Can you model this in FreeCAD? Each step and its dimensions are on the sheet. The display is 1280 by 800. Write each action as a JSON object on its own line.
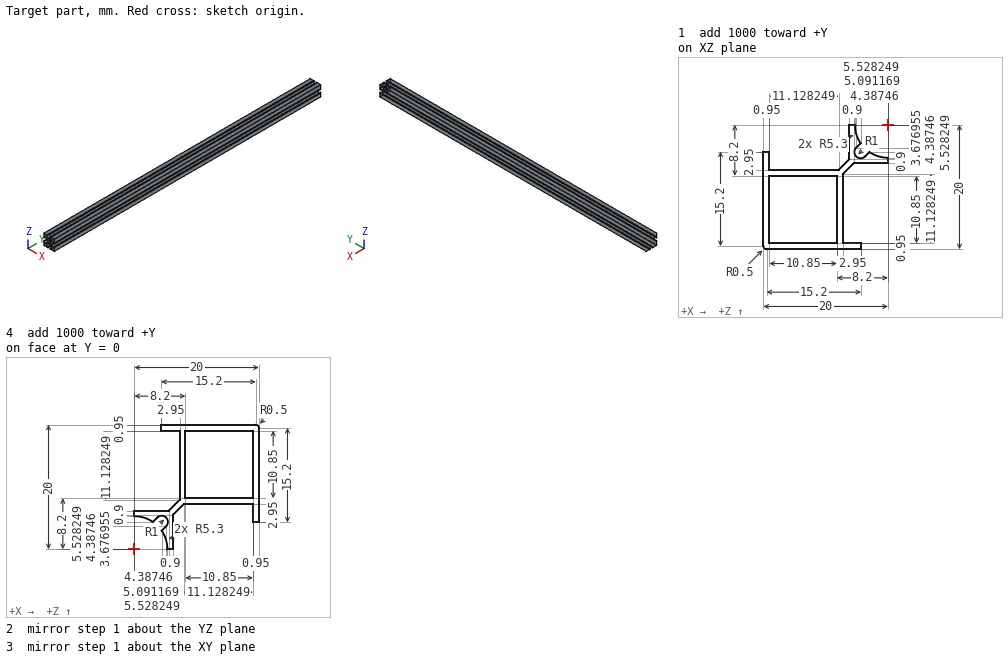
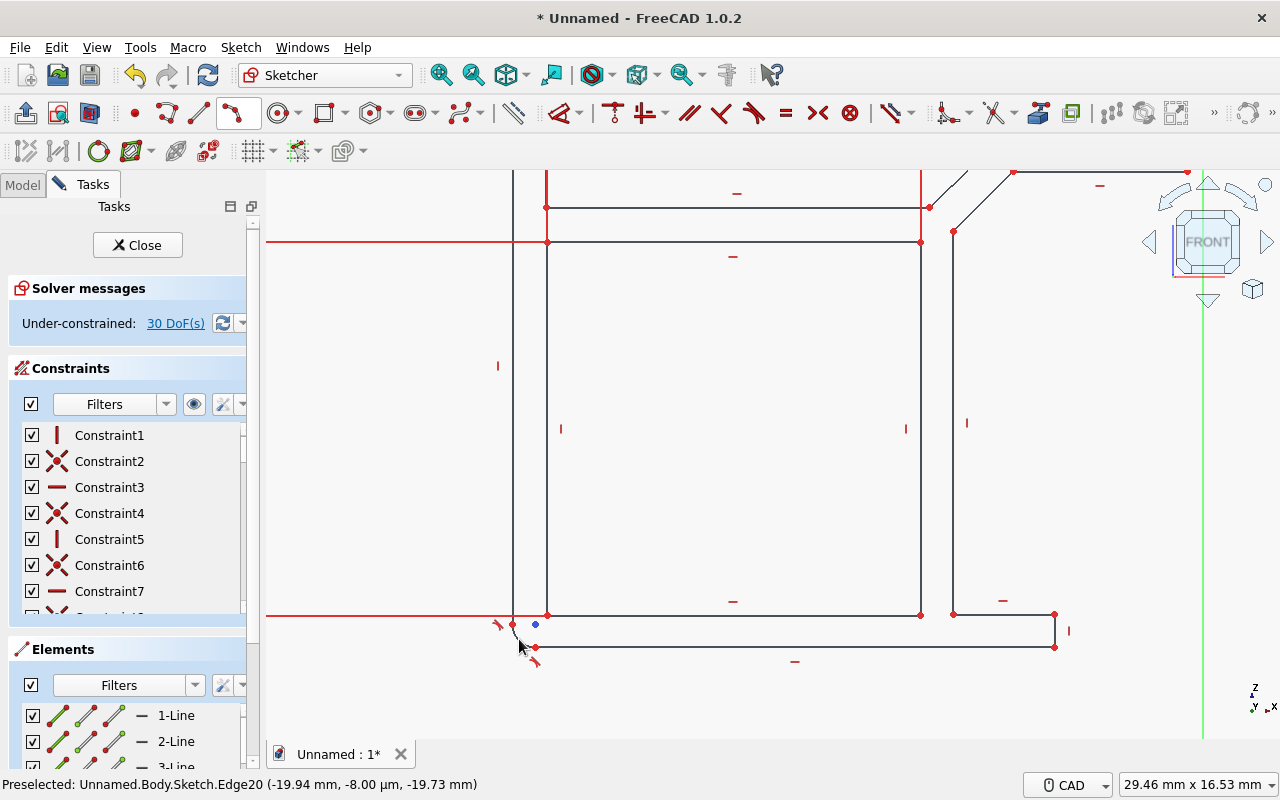
{"action": "scroll", "coordinate": [517, 641], "scroll_direction": "down", "scroll_amount": 3}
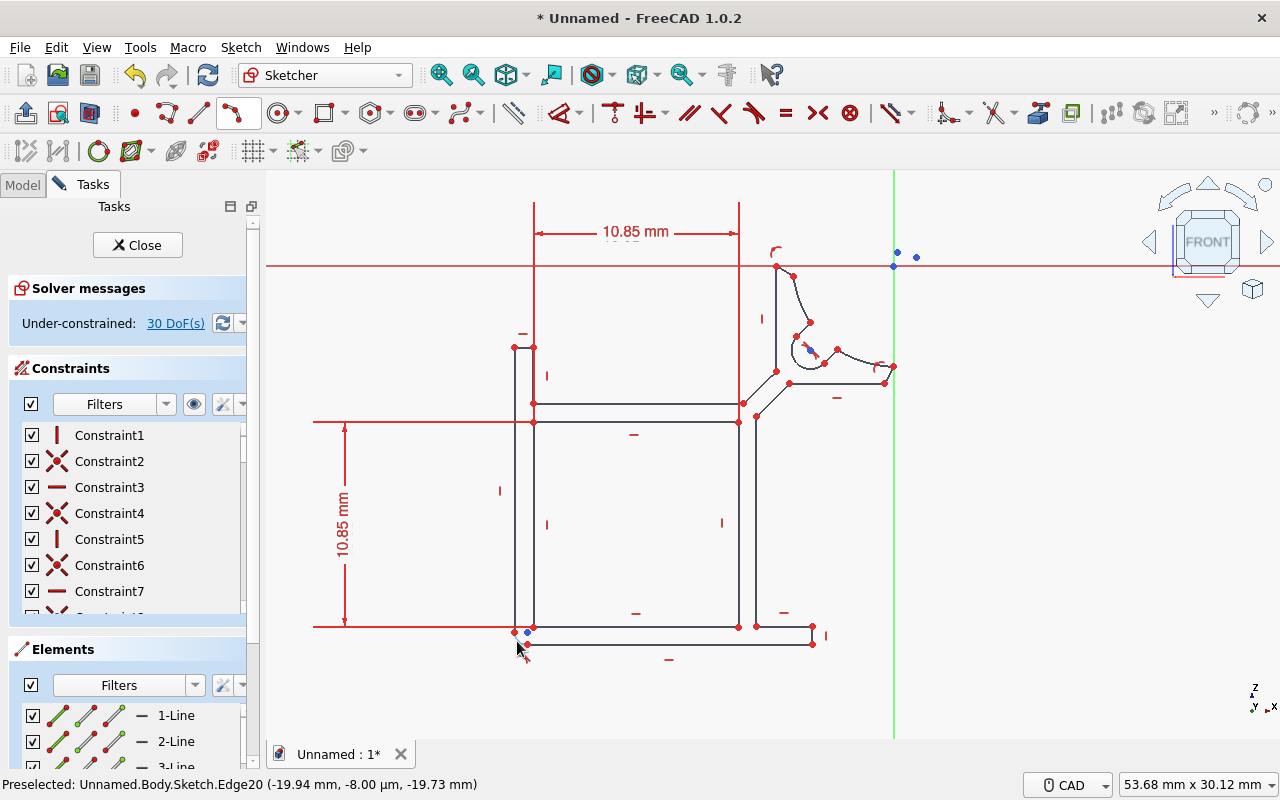
{"action": "scroll", "coordinate": [788, 273], "scroll_direction": "up", "scroll_amount": 5}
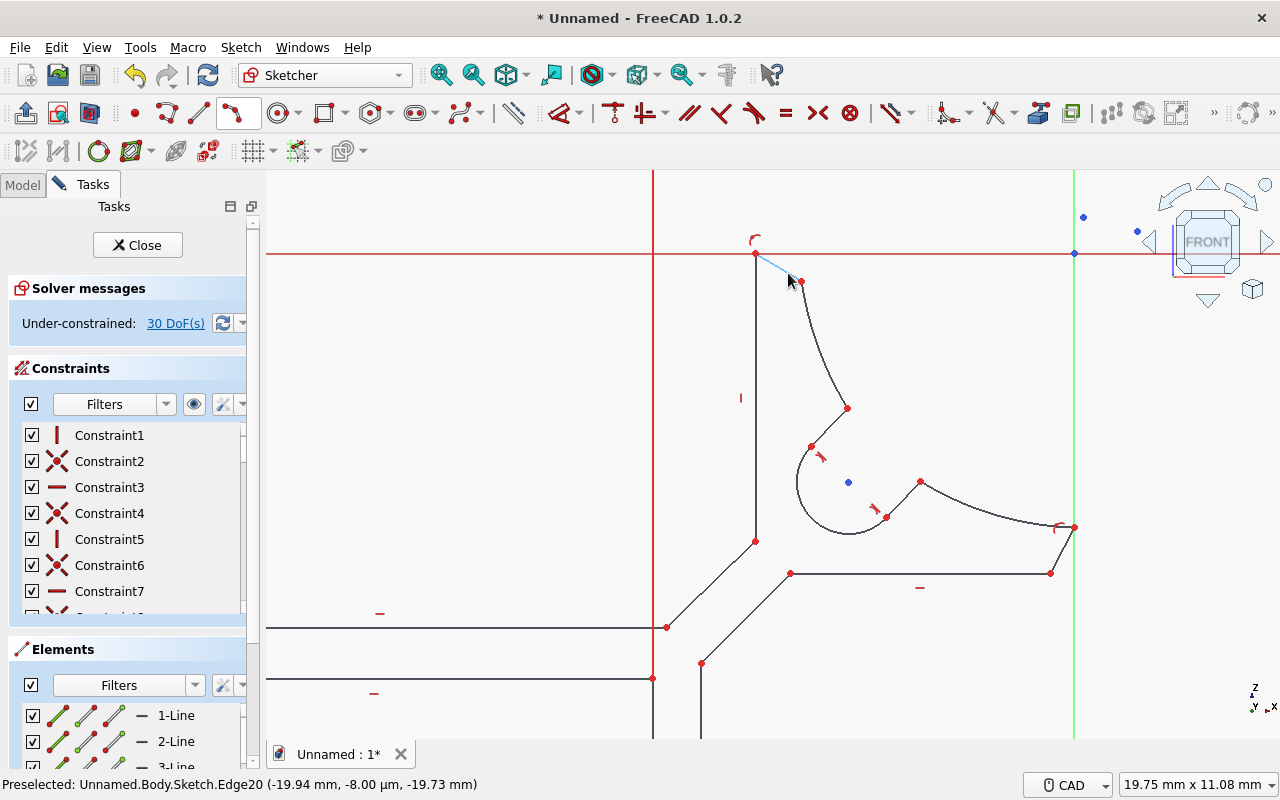
{"action": "left_click", "coordinate": [788, 273]}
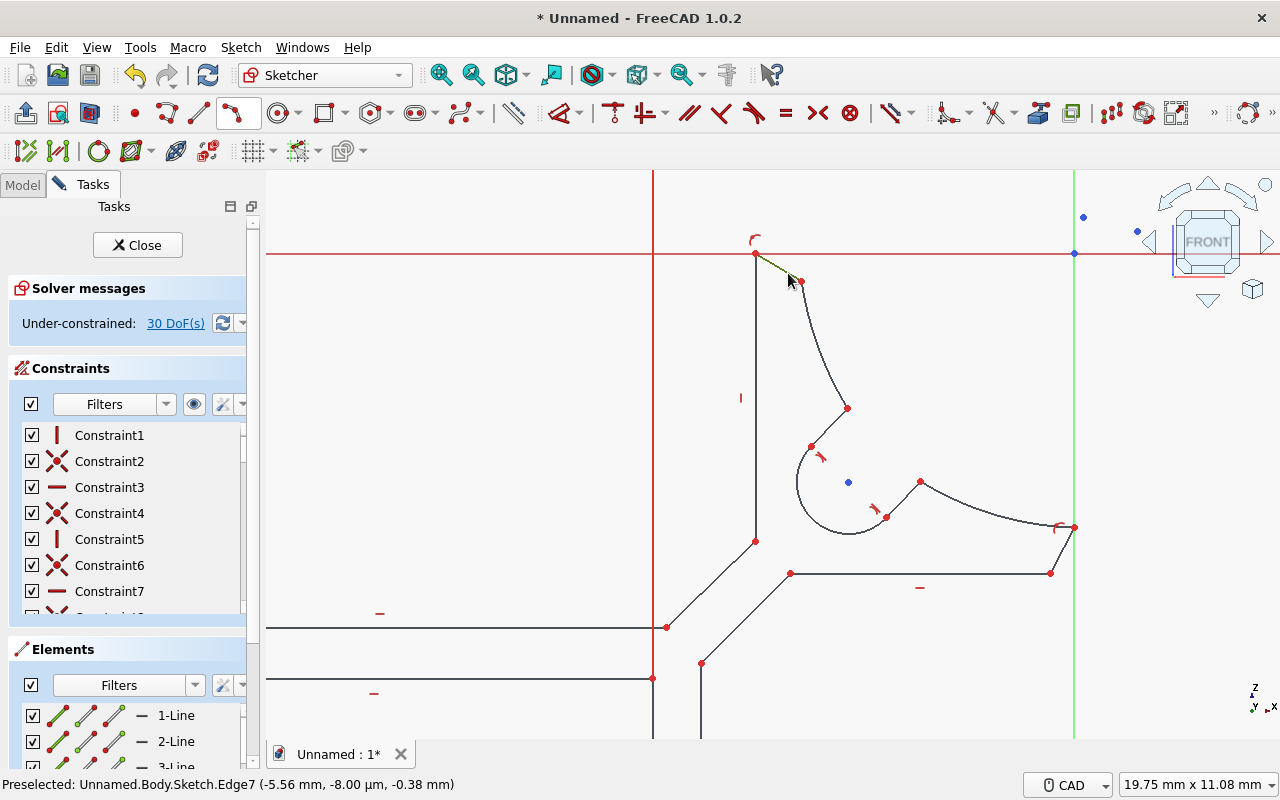
{"action": "left_click", "coordinate": [668, 114]}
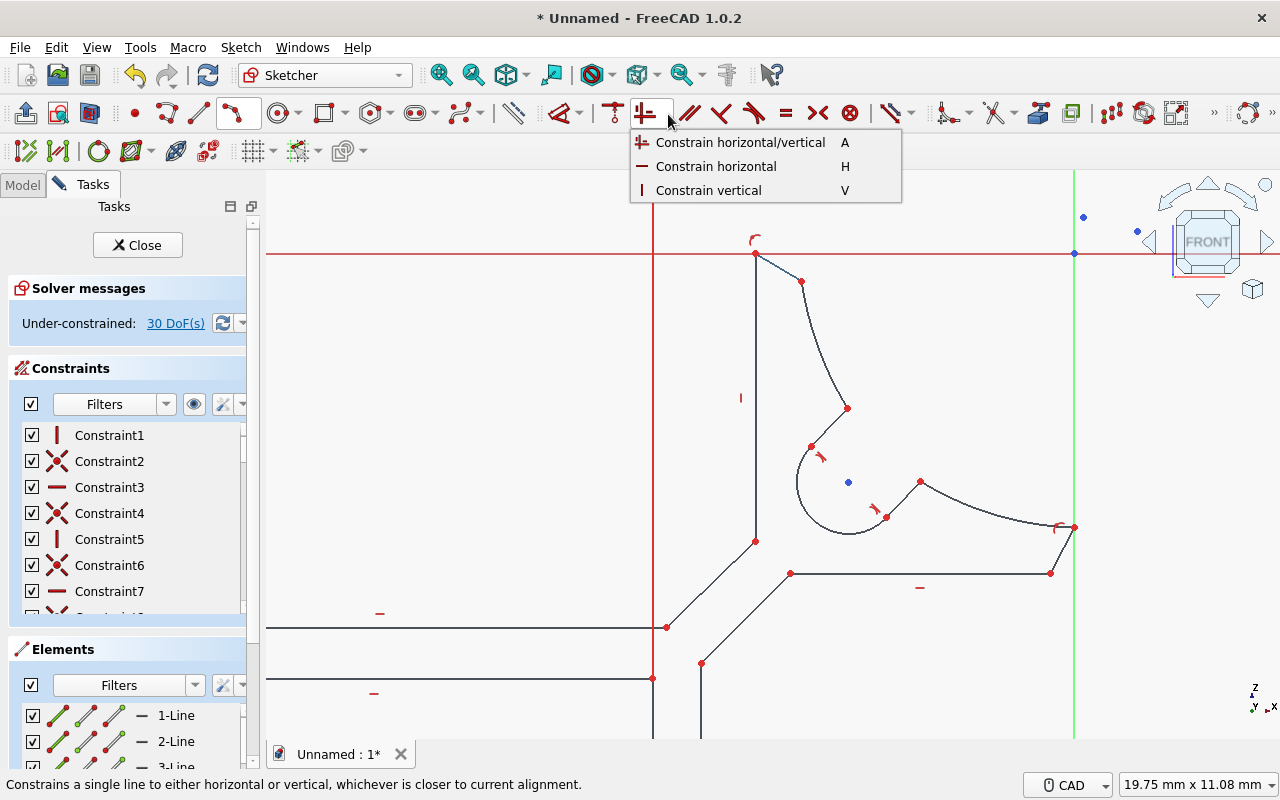
{"action": "left_click", "coordinate": [766, 166]}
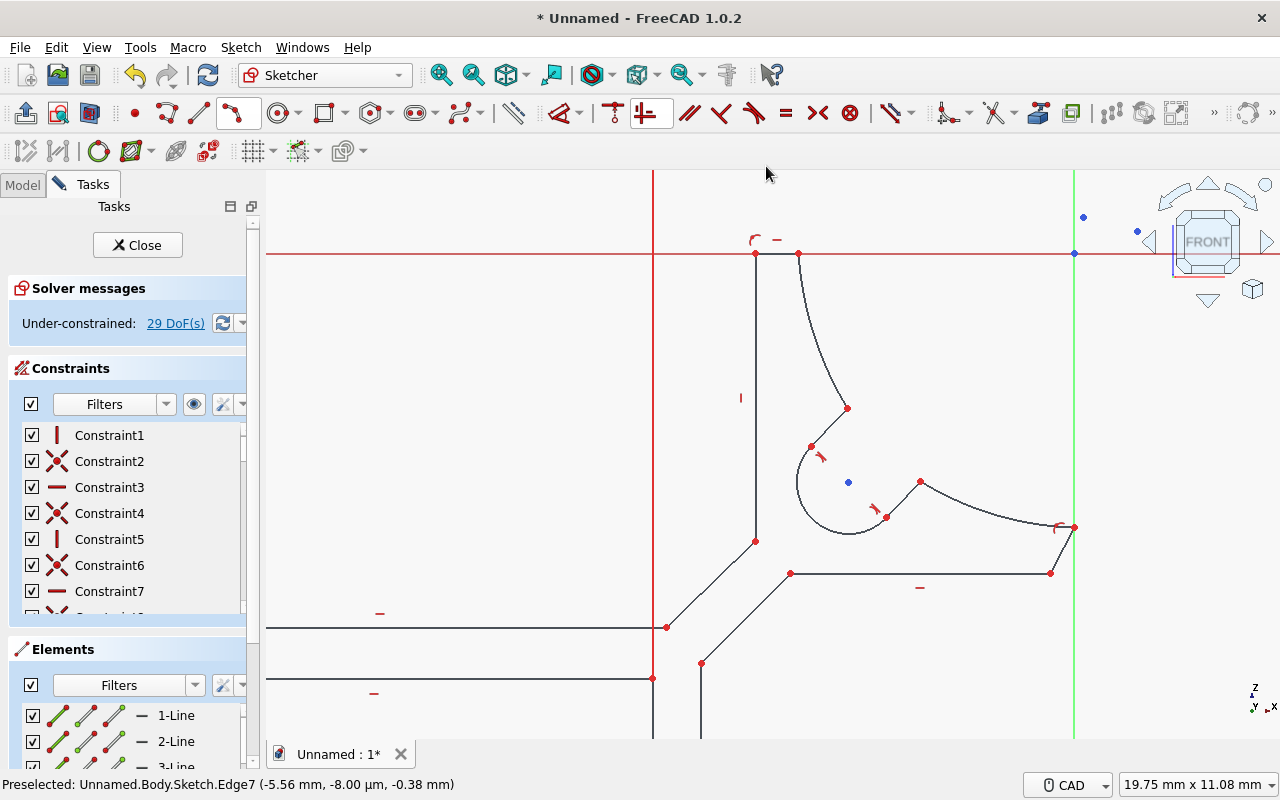
{"action": "left_click", "coordinate": [1058, 560]}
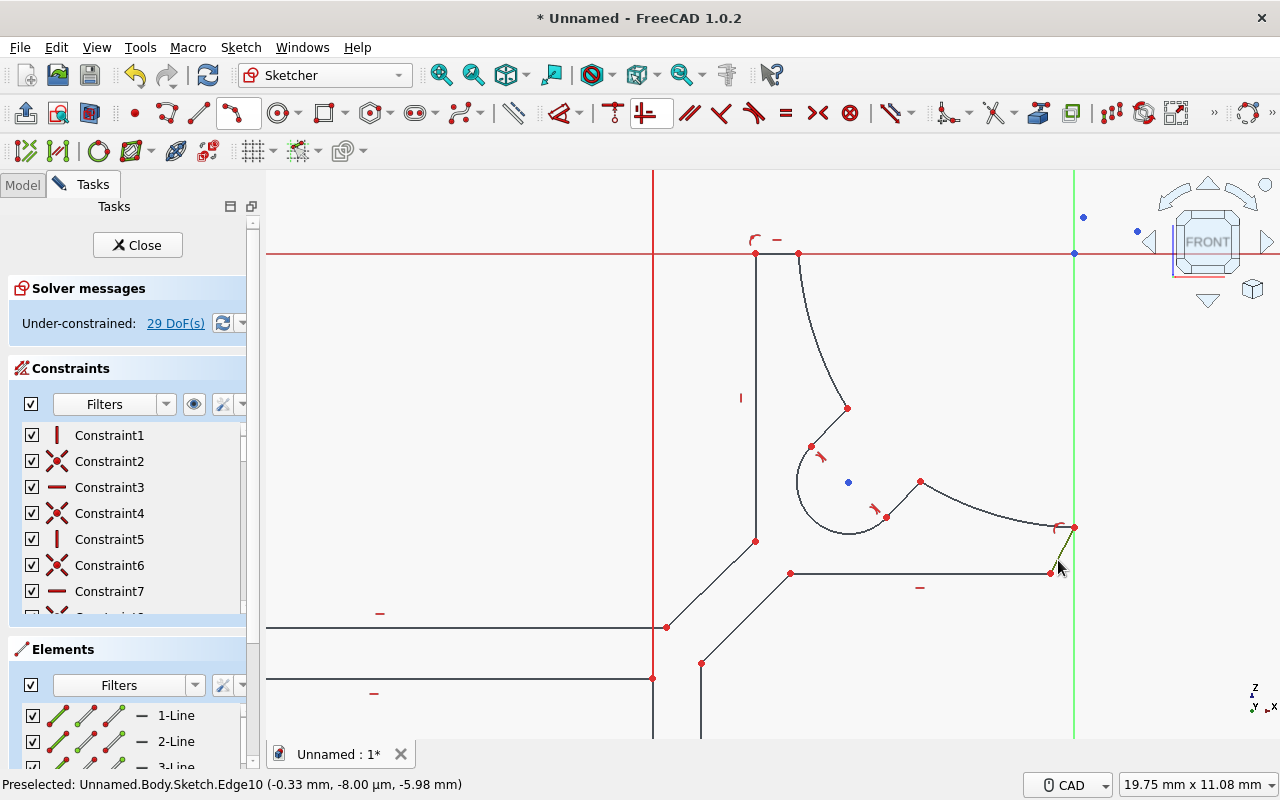
{"action": "key", "text": "v"}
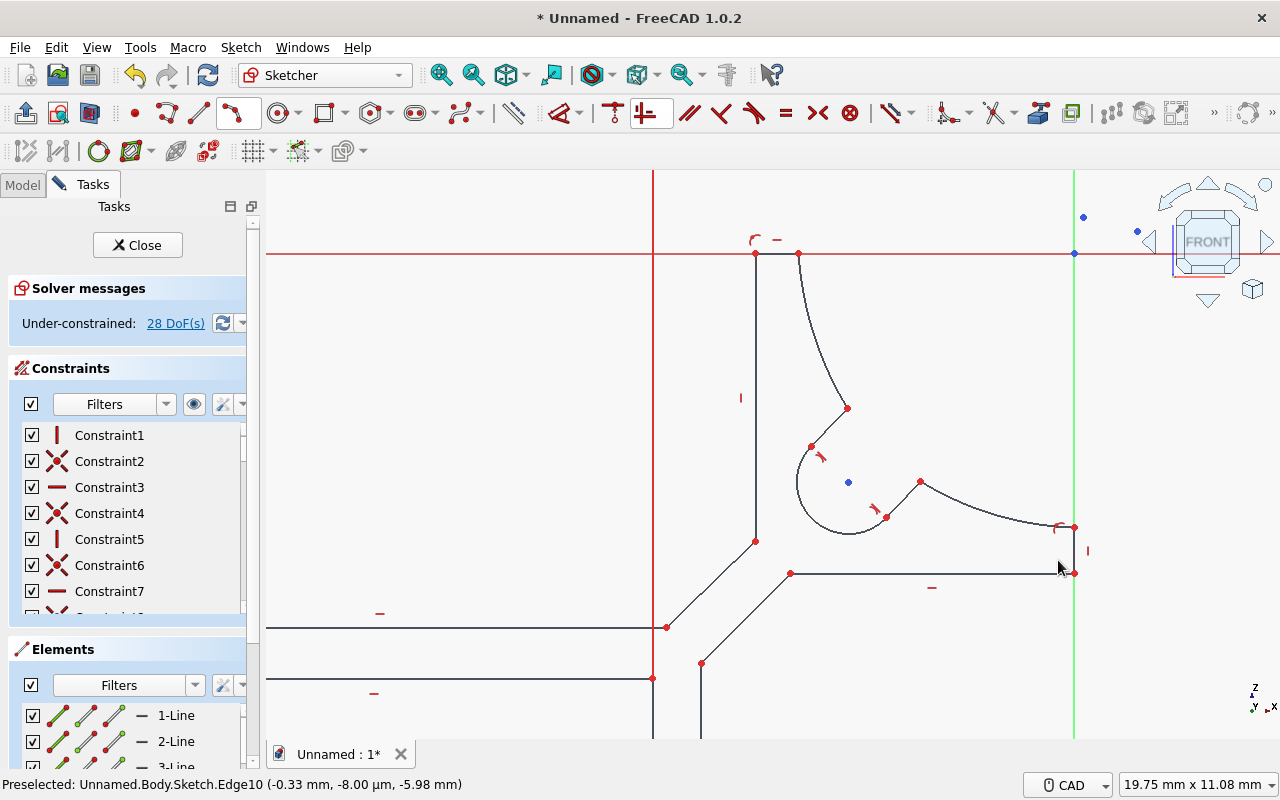
{"action": "left_click", "coordinate": [805, 302]}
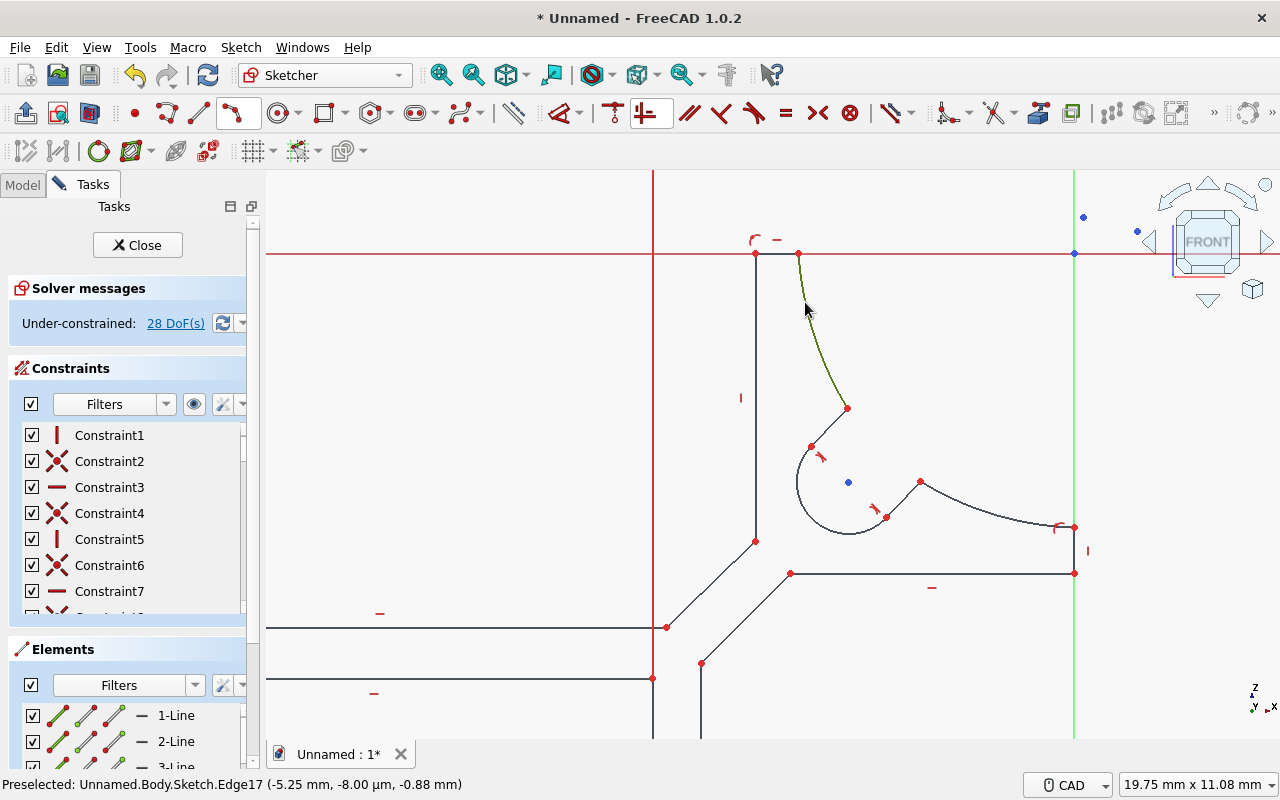
{"action": "left_click", "coordinate": [964, 504]}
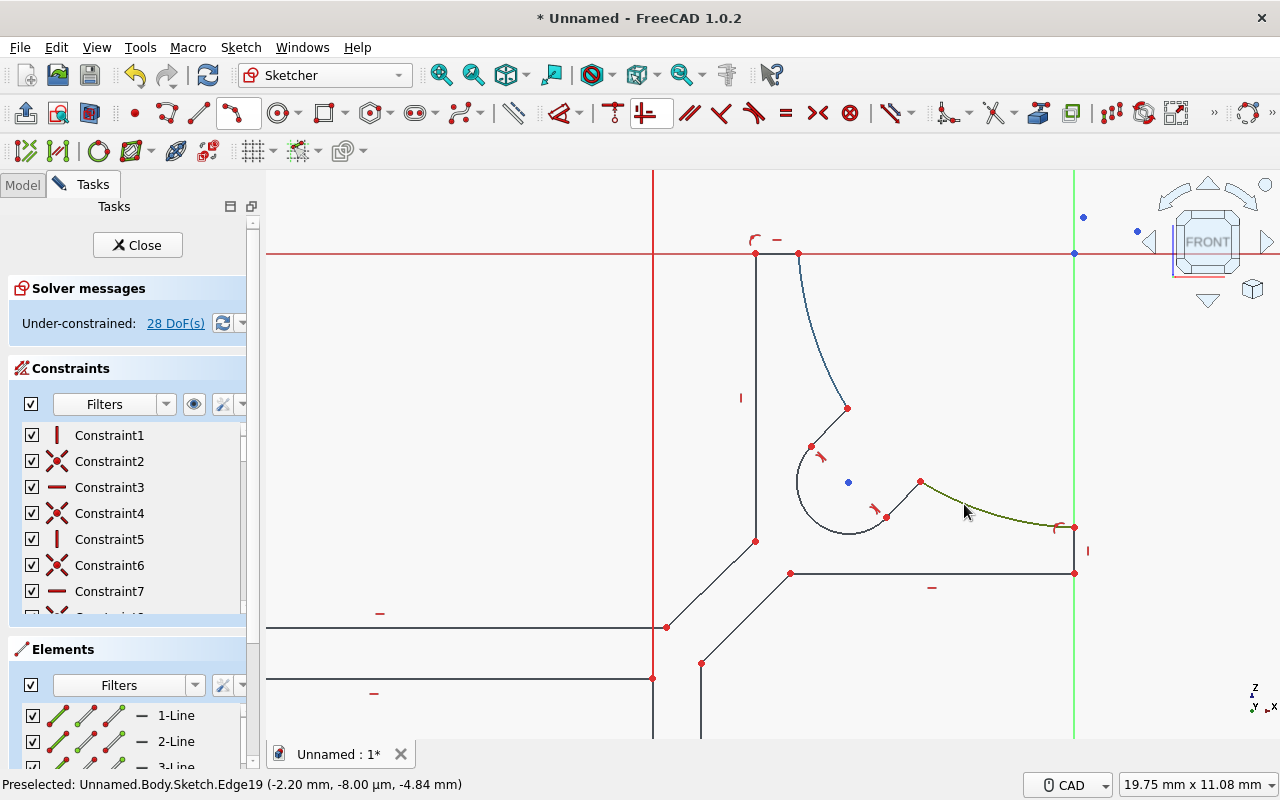
{"action": "left_click", "coordinate": [614, 114]}